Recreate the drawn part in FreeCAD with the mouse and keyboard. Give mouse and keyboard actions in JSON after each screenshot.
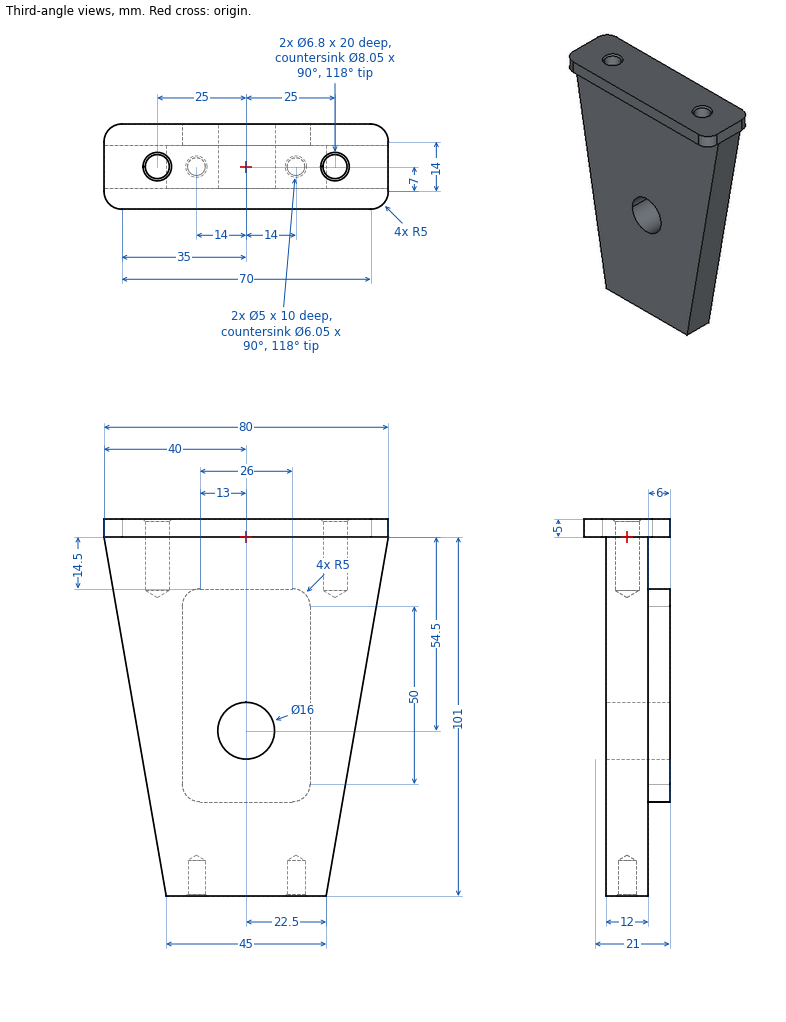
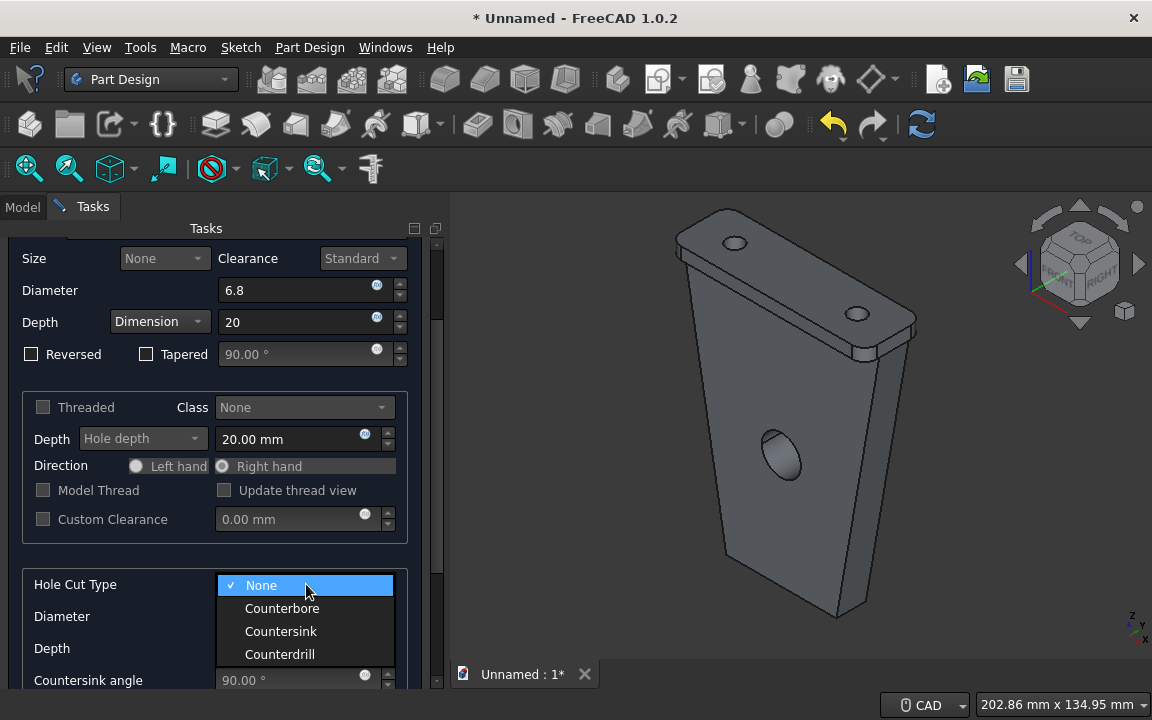
{"action": "left_click", "coordinate": [304, 632]}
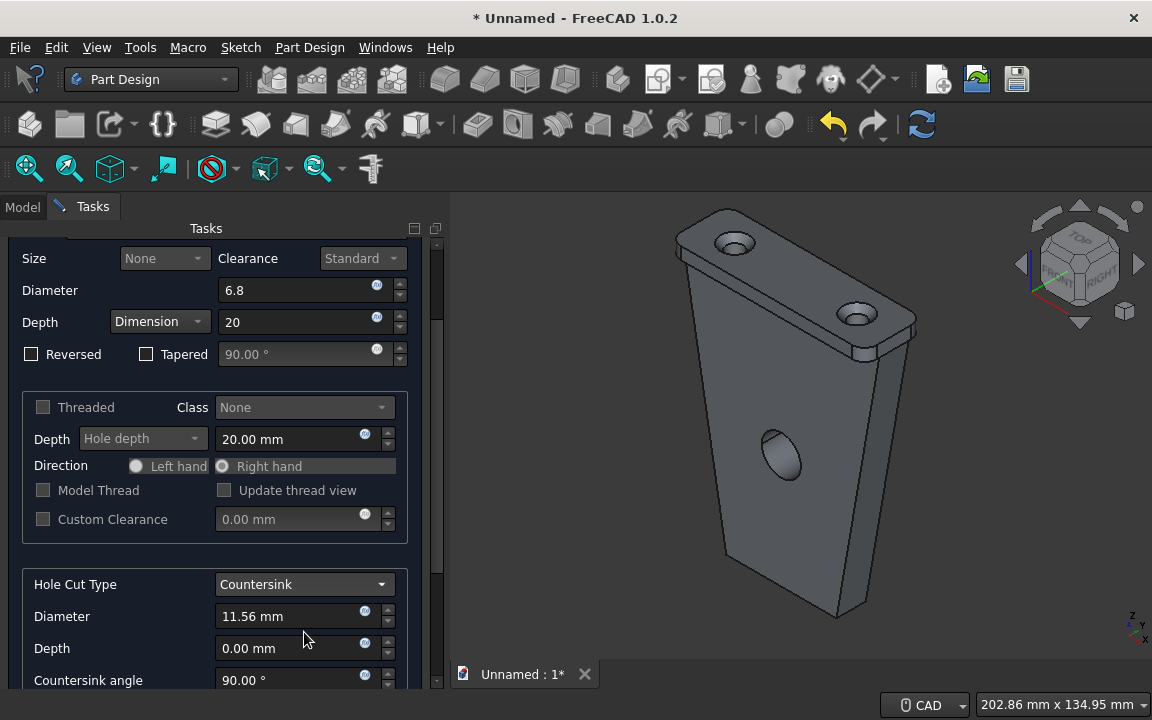
{"action": "triple_click", "coordinate": [298, 616]}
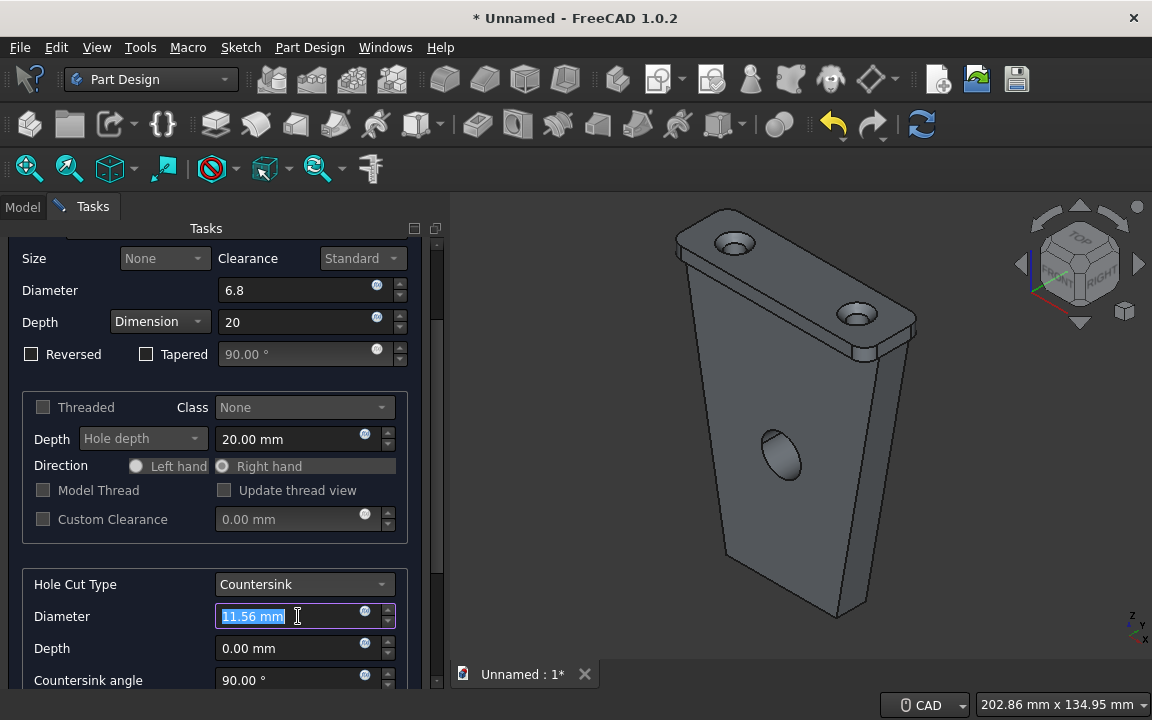
{"action": "type", "text": "8.05"}
{"action": "key", "text": "Tab"}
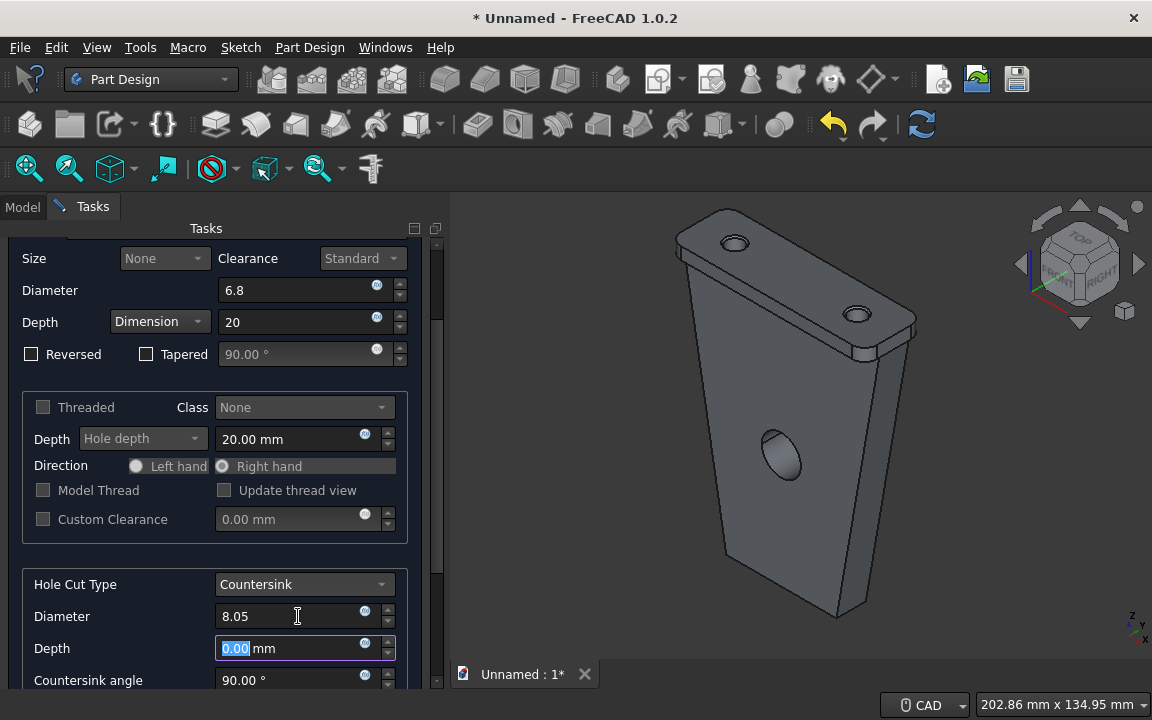
{"action": "scroll", "coordinate": [437, 463], "scroll_direction": "up", "scroll_amount": 3}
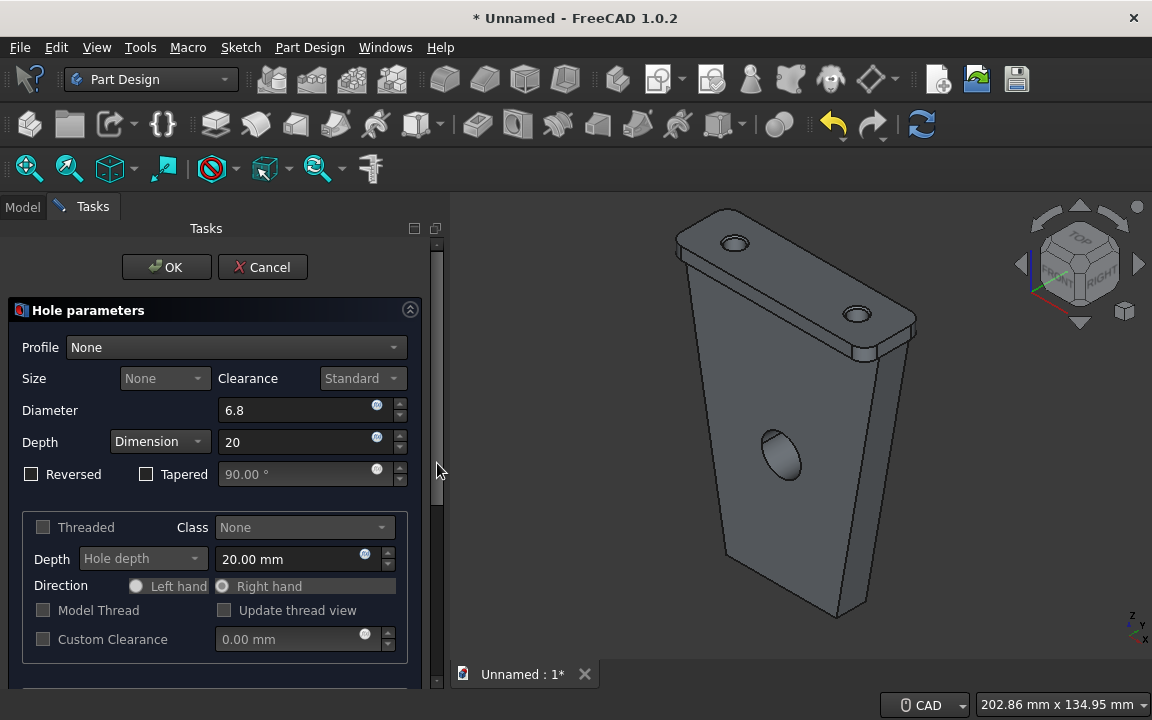
{"action": "left_click", "coordinate": [167, 267]}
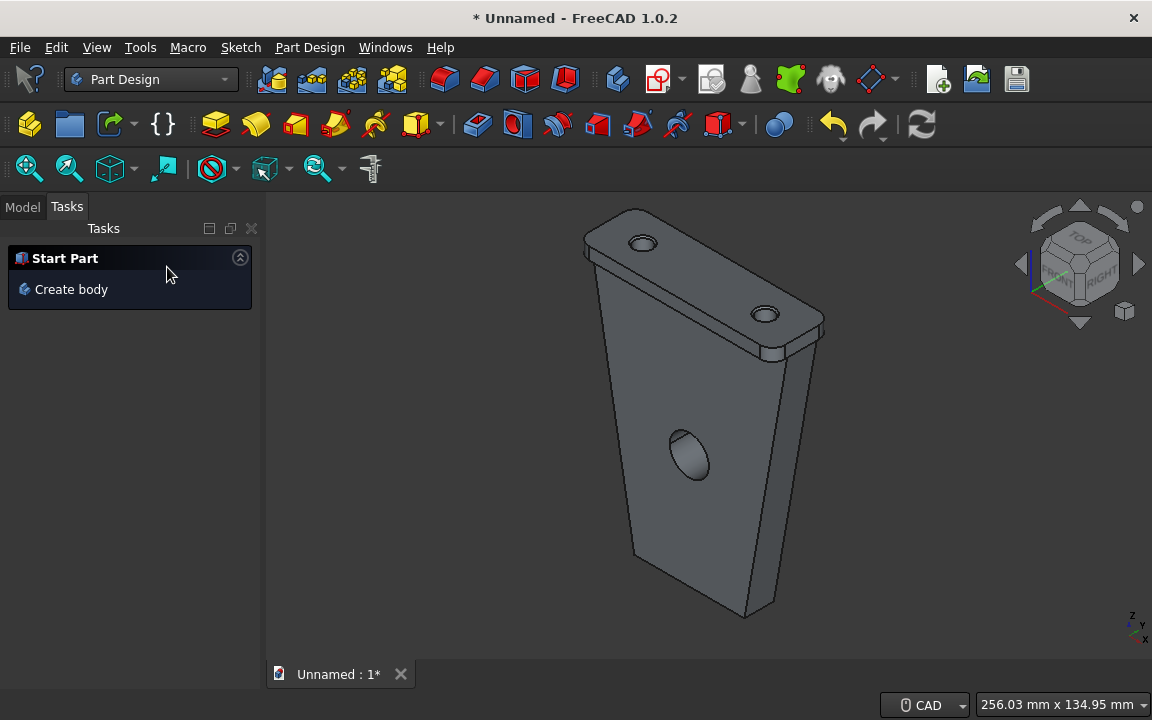
{"action": "key", "text": "5"}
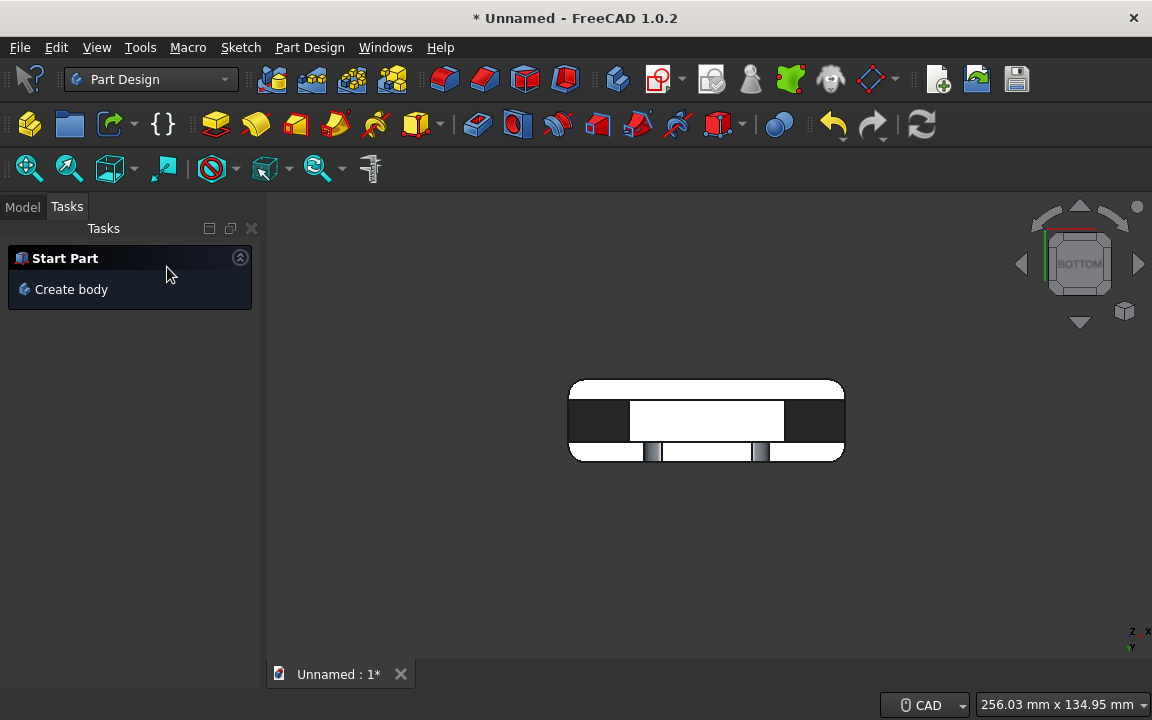
{"action": "left_click", "coordinate": [30, 170]}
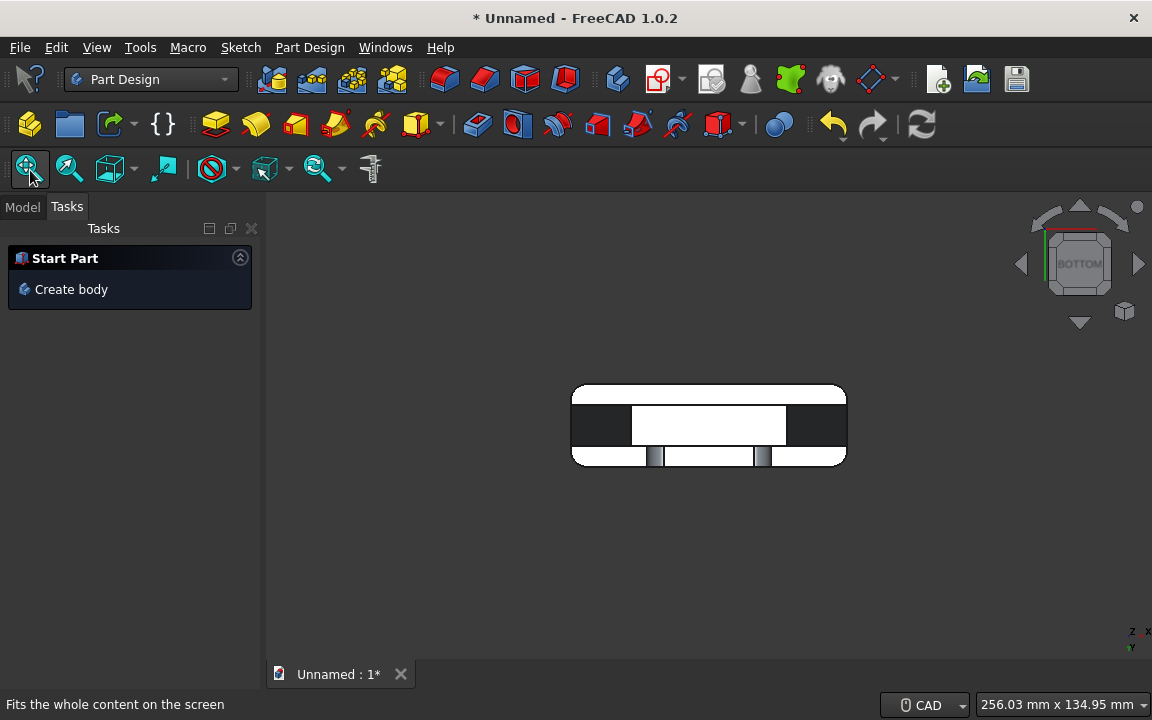
{"action": "left_click", "coordinate": [753, 424]}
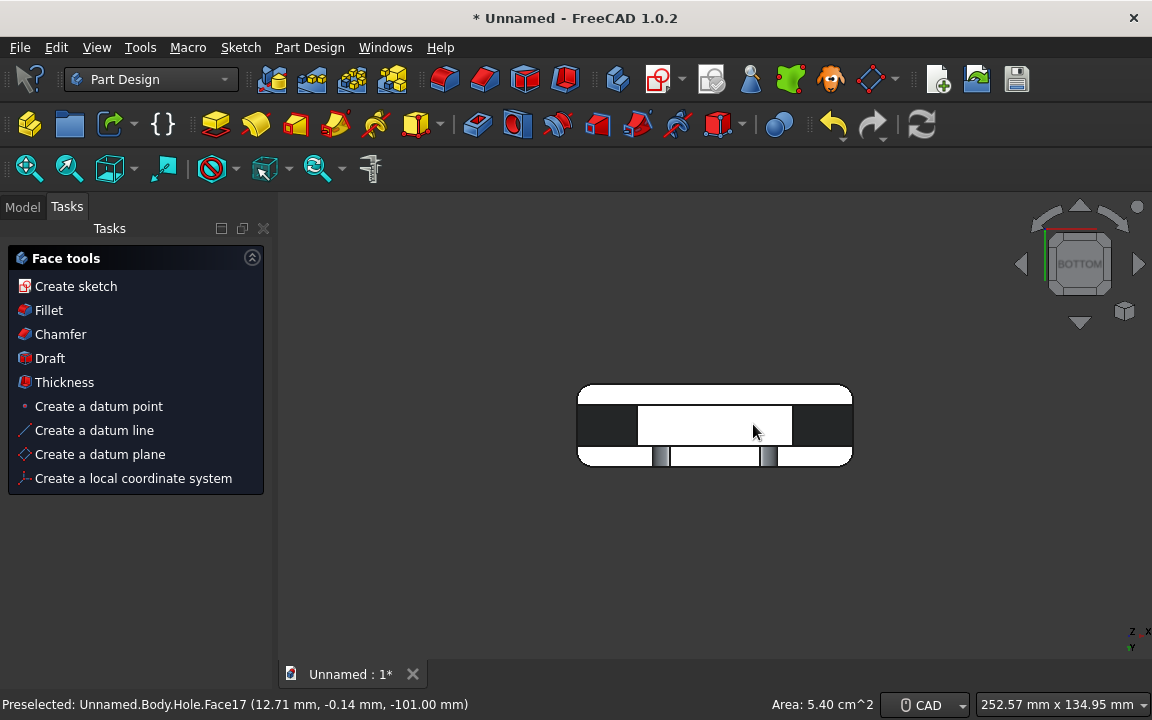
{"action": "left_click", "coordinate": [658, 80]}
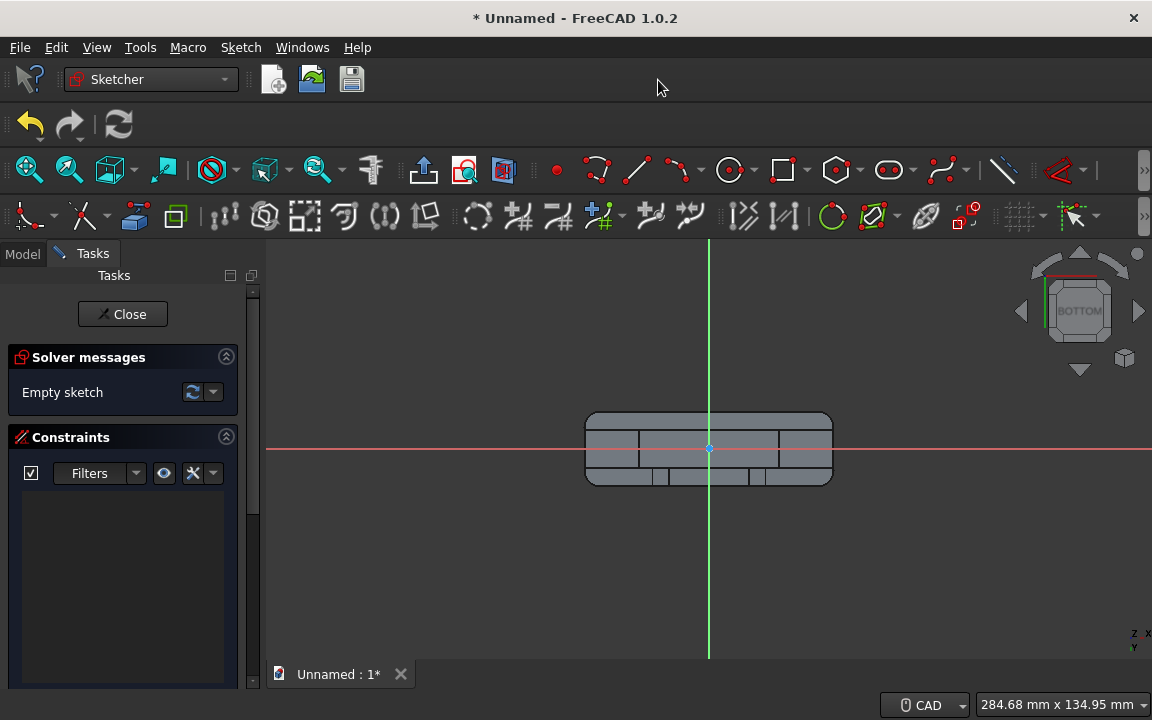
{"action": "scroll", "coordinate": [726, 449], "scroll_direction": "up", "scroll_amount": 8}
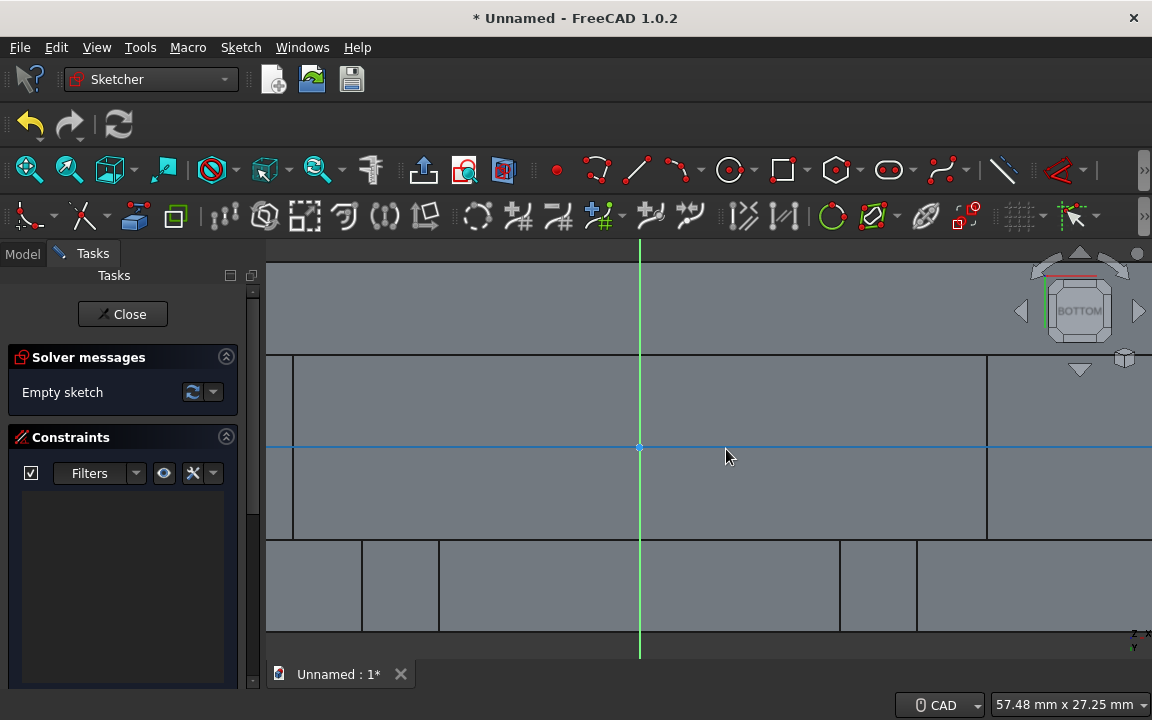
{"action": "left_click", "coordinate": [730, 170]}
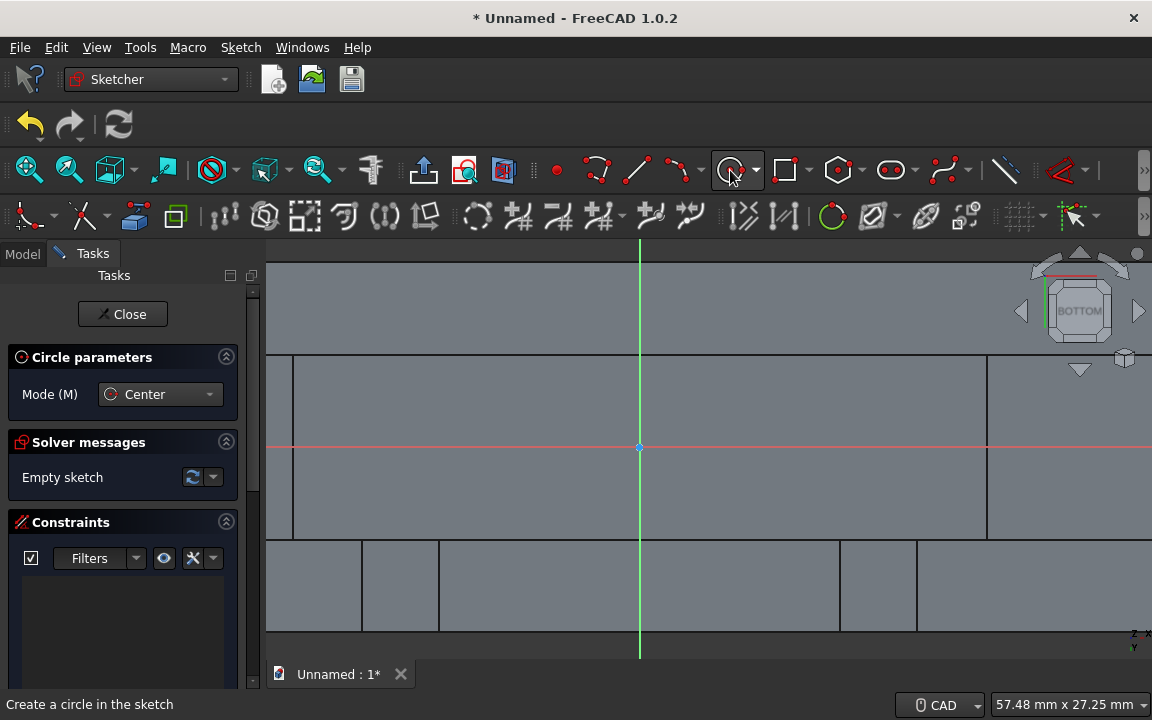
{"action": "left_click", "coordinate": [856, 447]}
{"action": "mouse_move", "coordinate": [883, 420]}